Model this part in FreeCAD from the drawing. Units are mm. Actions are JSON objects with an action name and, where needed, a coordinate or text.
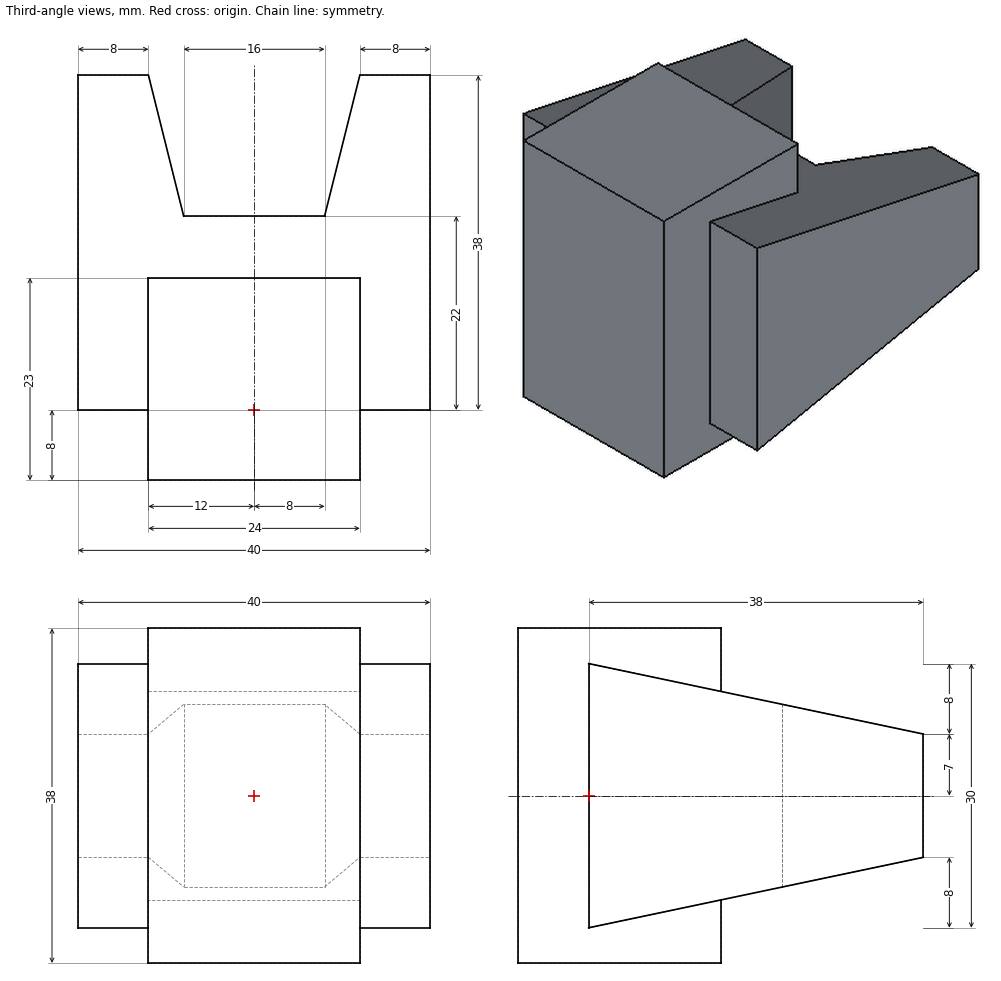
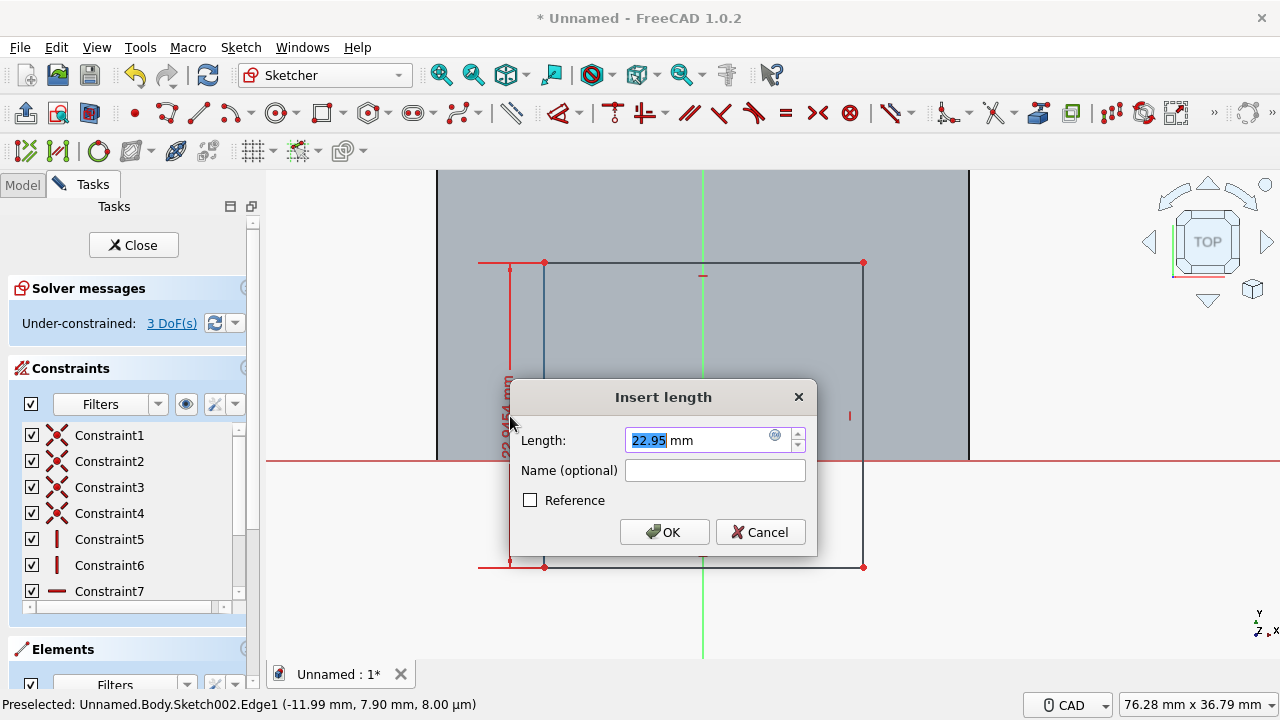
{"action": "type", "text": "23"}
{"action": "key", "text": "Return"}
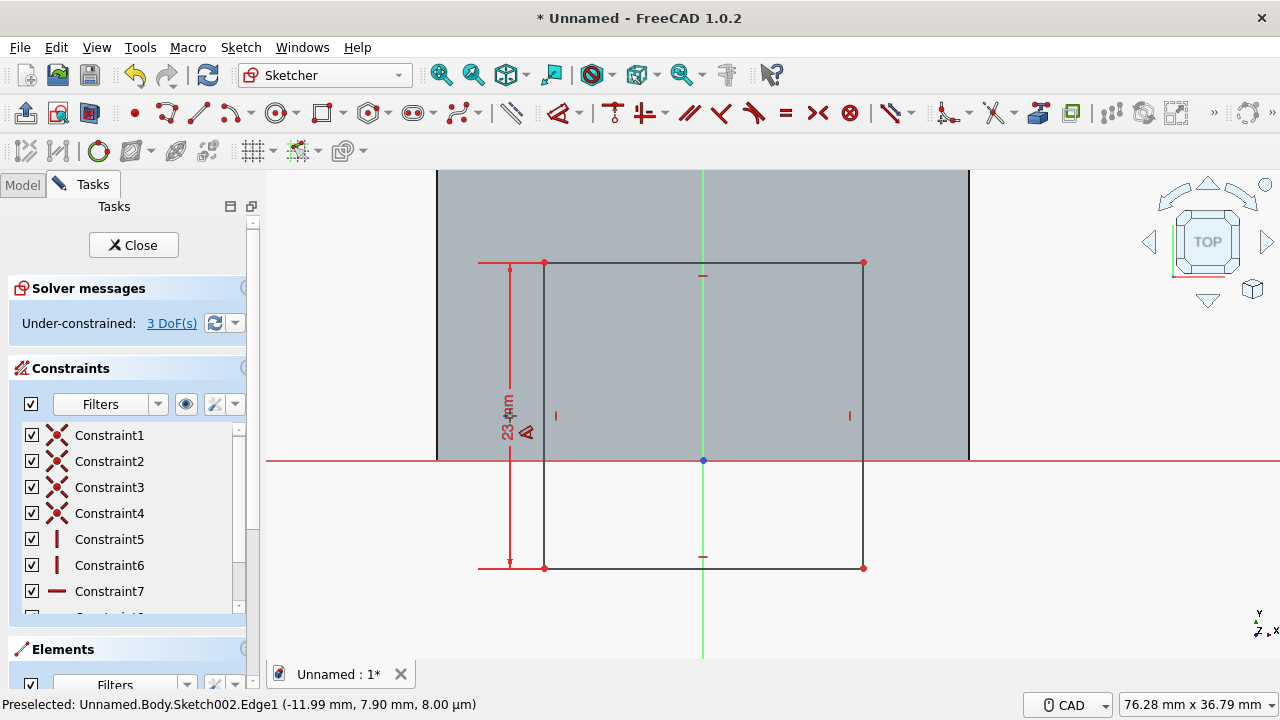
{"action": "left_click", "coordinate": [640, 569]}
{"action": "left_click", "coordinate": [630, 603]}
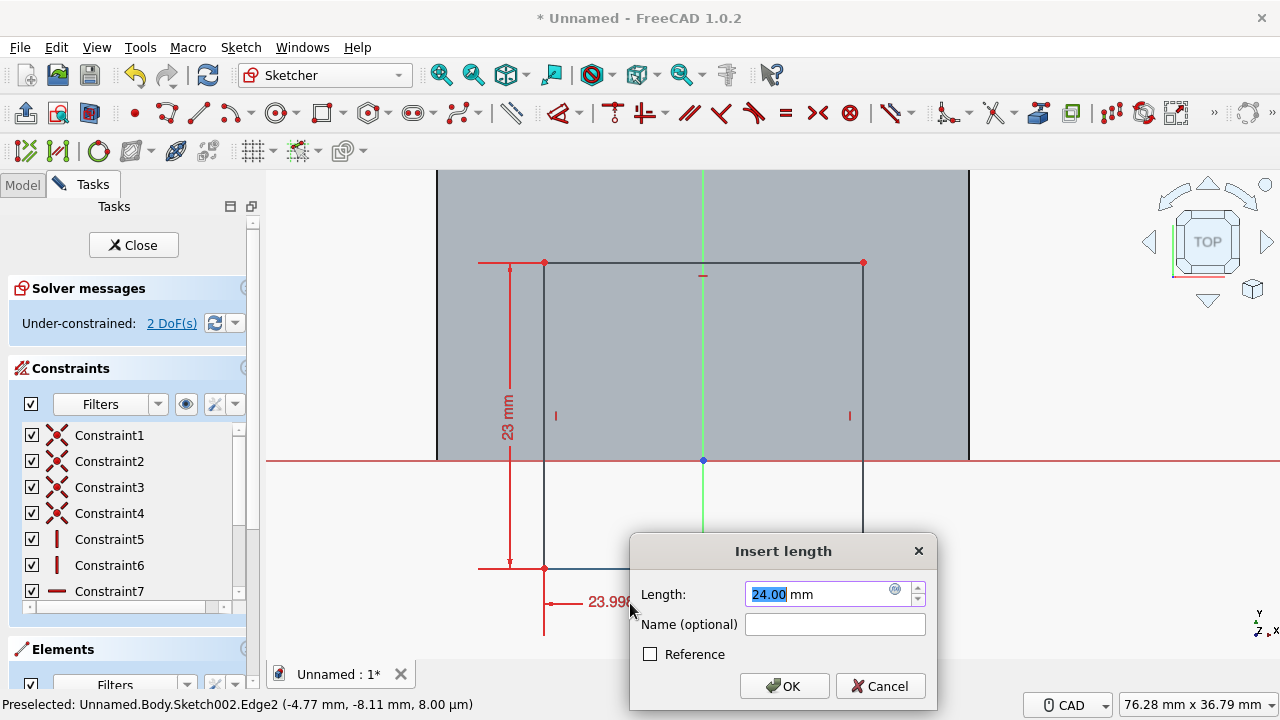
{"action": "type", "text": "24"}
{"action": "key", "text": "Return"}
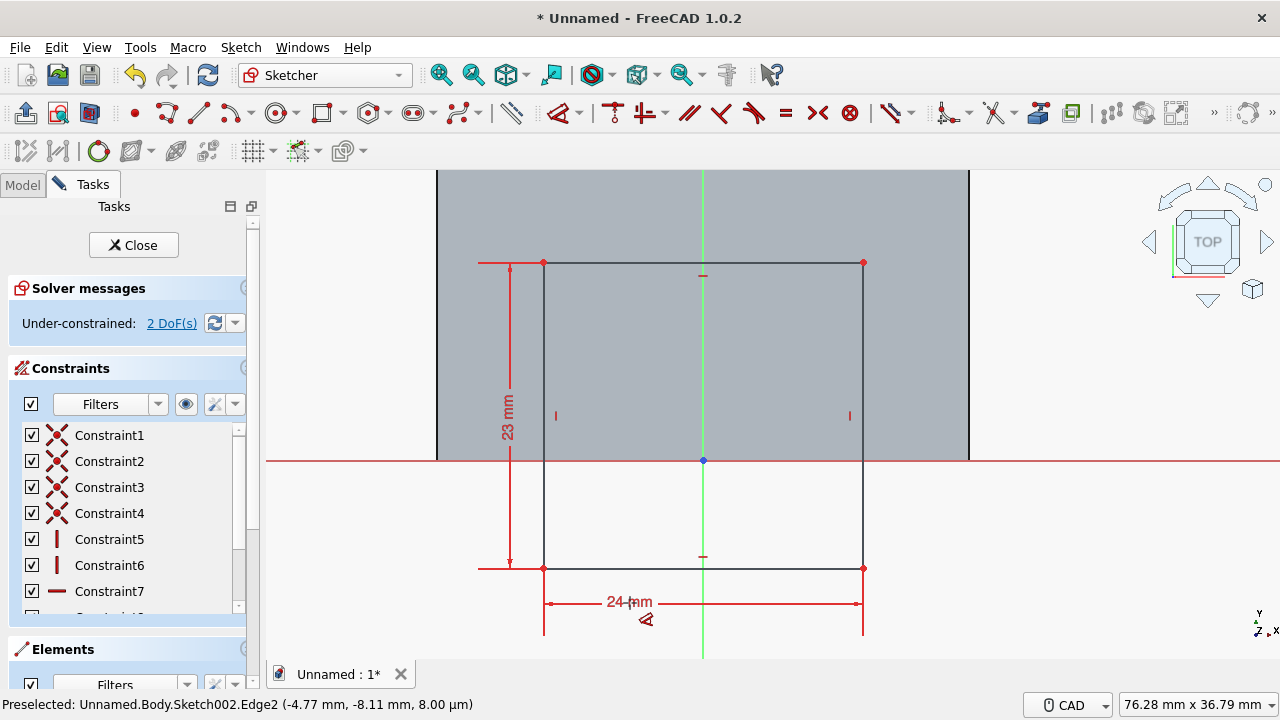
{"action": "left_click", "coordinate": [544, 569]}
{"action": "left_click", "coordinate": [510, 515]}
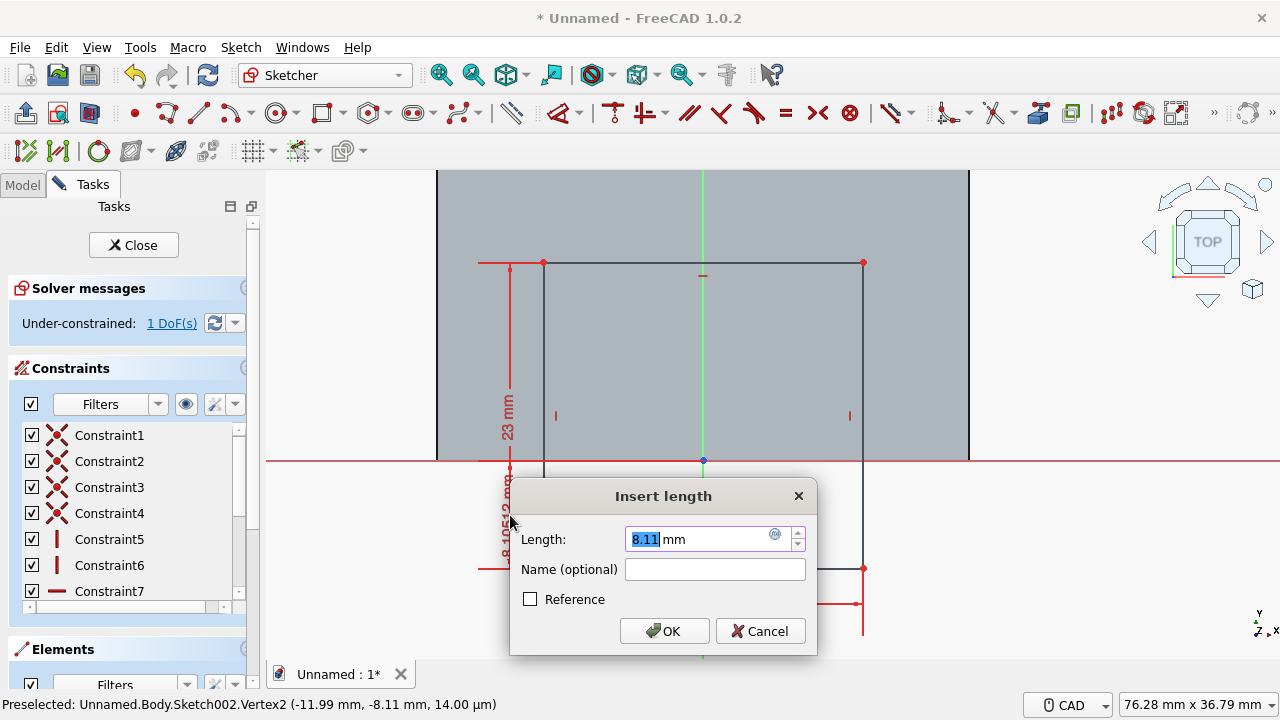
{"action": "type", "text": "8"}
{"action": "key", "text": "Return"}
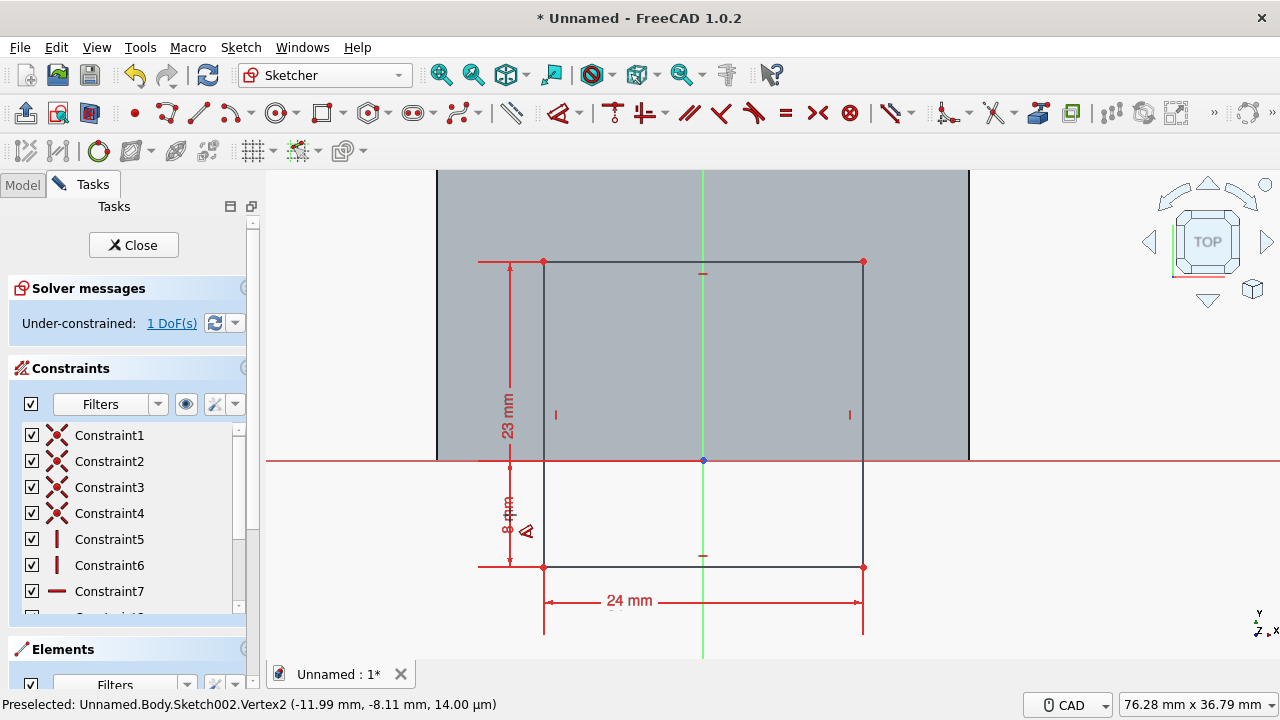
{"action": "left_click", "coordinate": [544, 262]}
{"action": "left_click", "coordinate": [624, 228]}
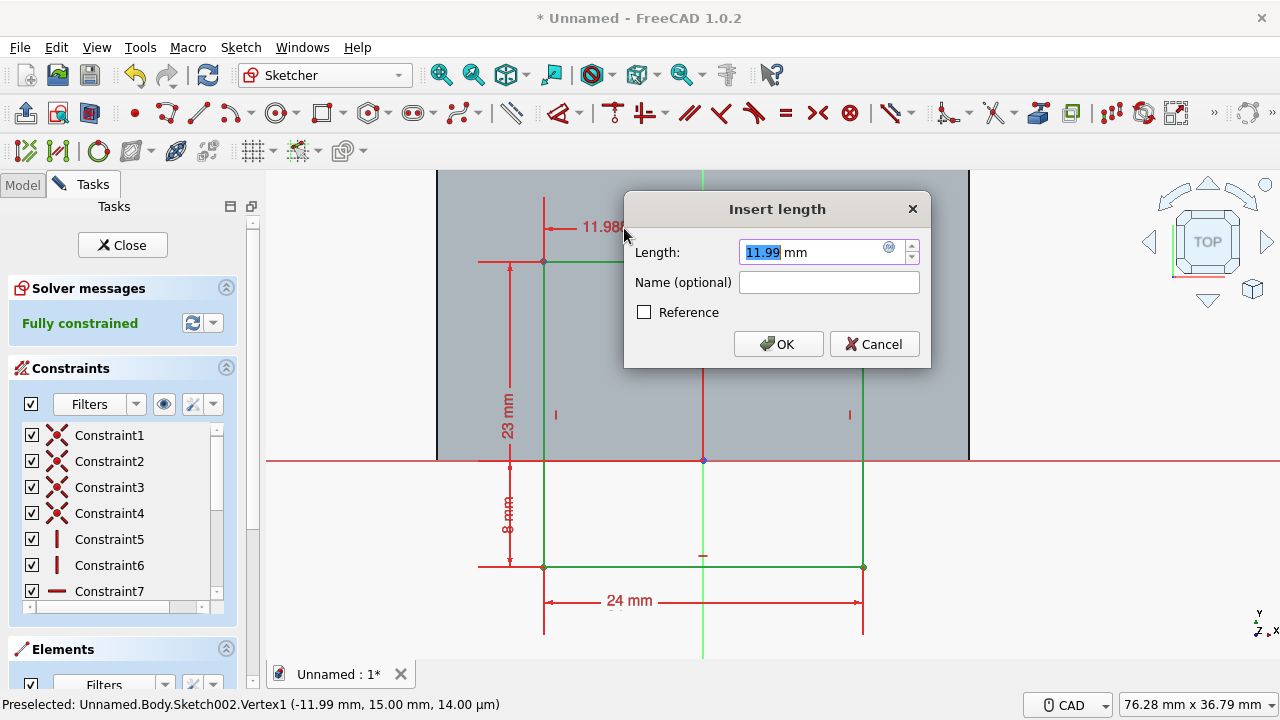
{"action": "type", "text": "12"}
{"action": "key", "text": "Return"}
{"action": "key", "text": "Escape"}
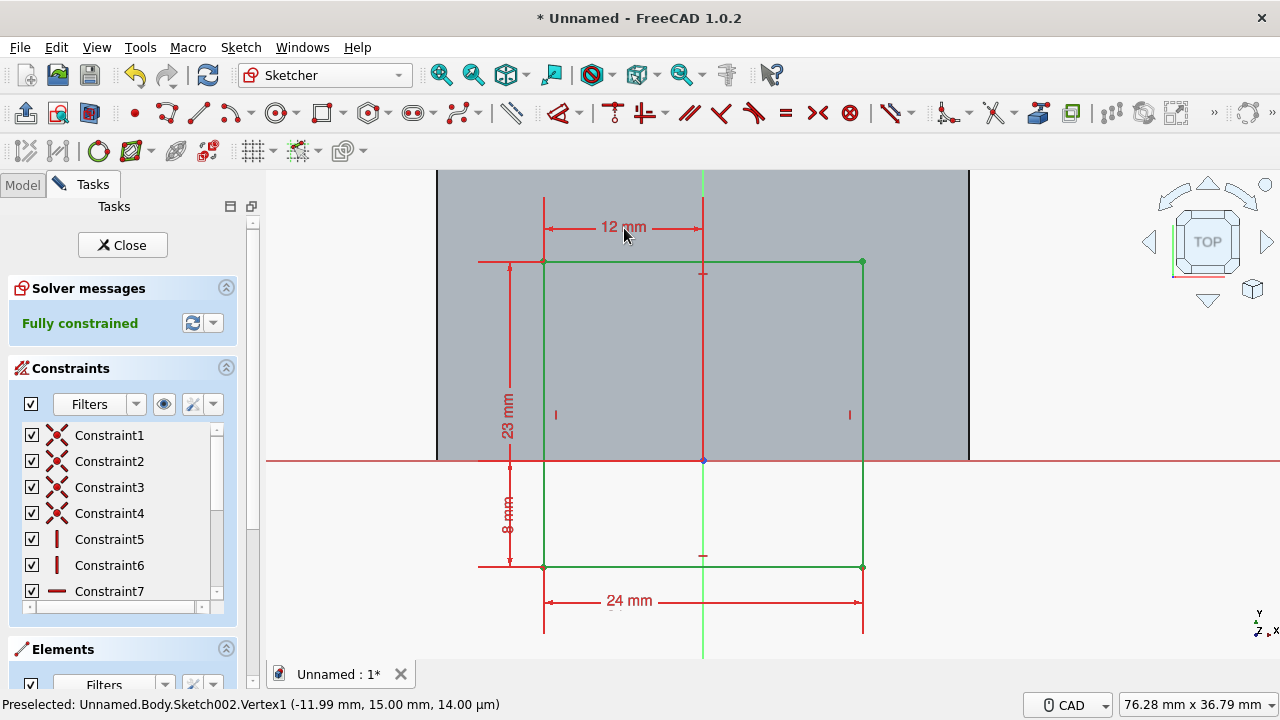
{"action": "left_click", "coordinate": [123, 245]}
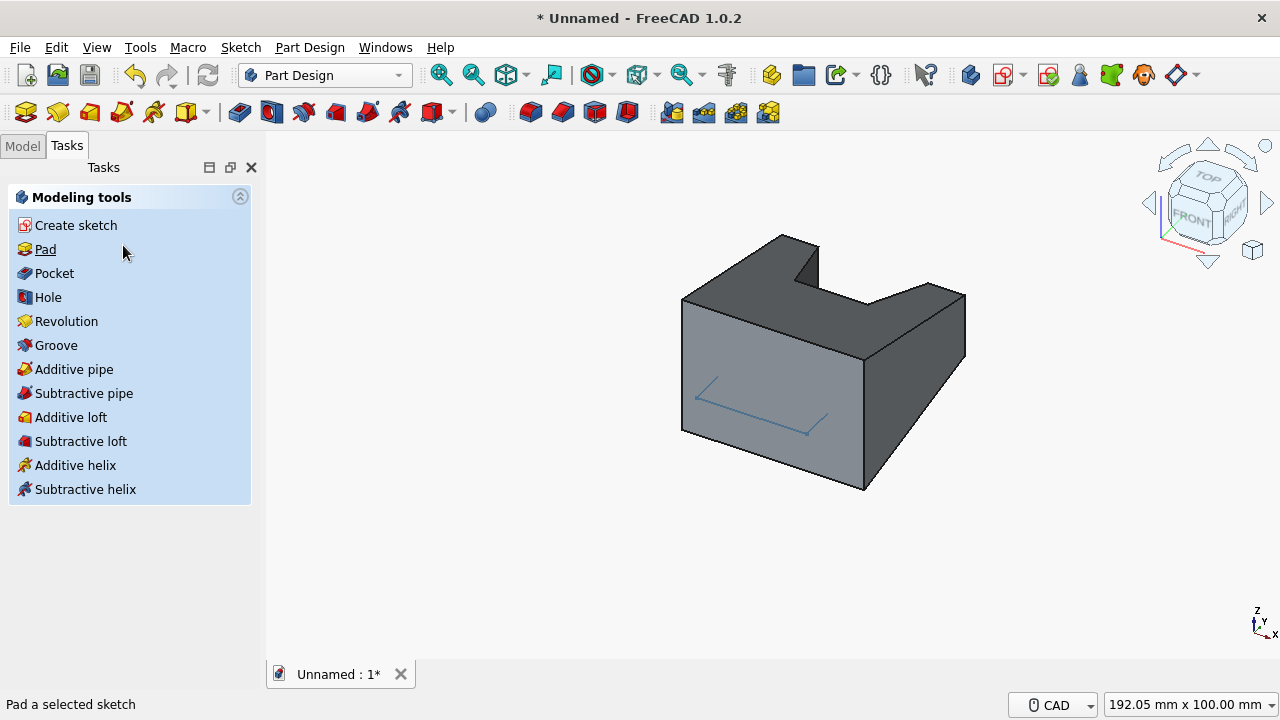
{"action": "left_click", "coordinate": [26, 112]}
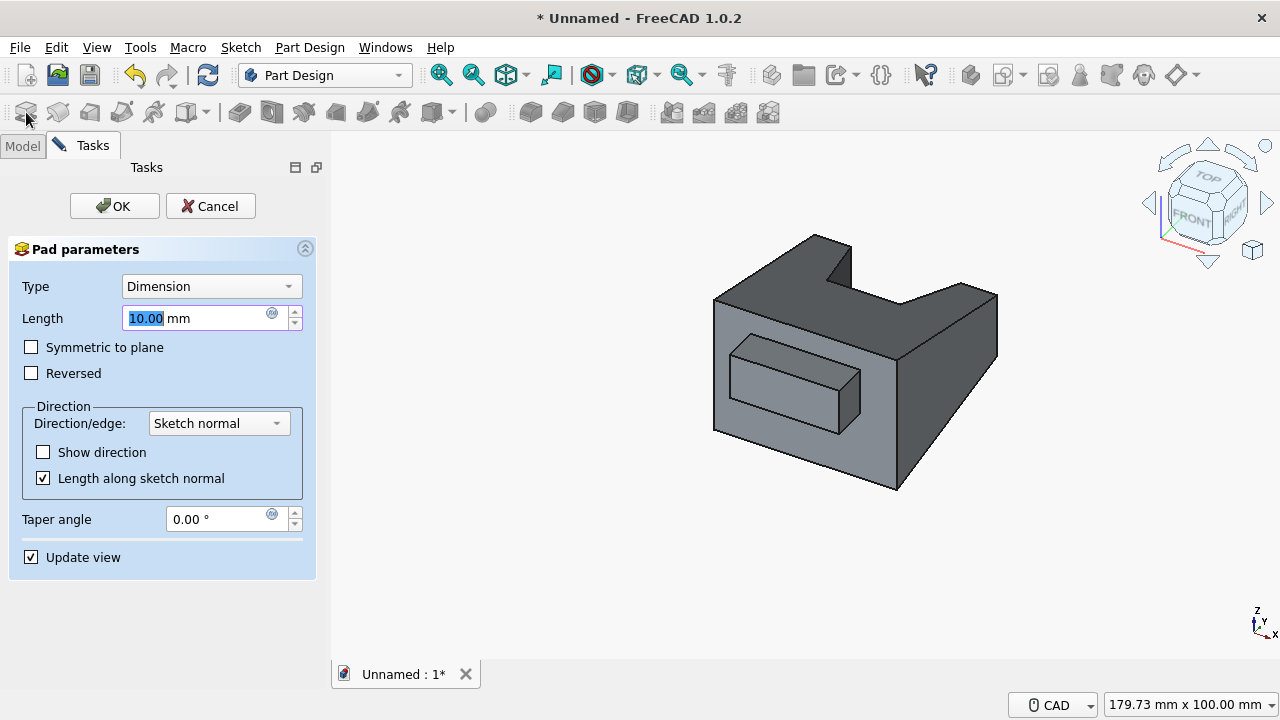
{"action": "type", "text": "38"}
{"action": "key", "text": "Tab"}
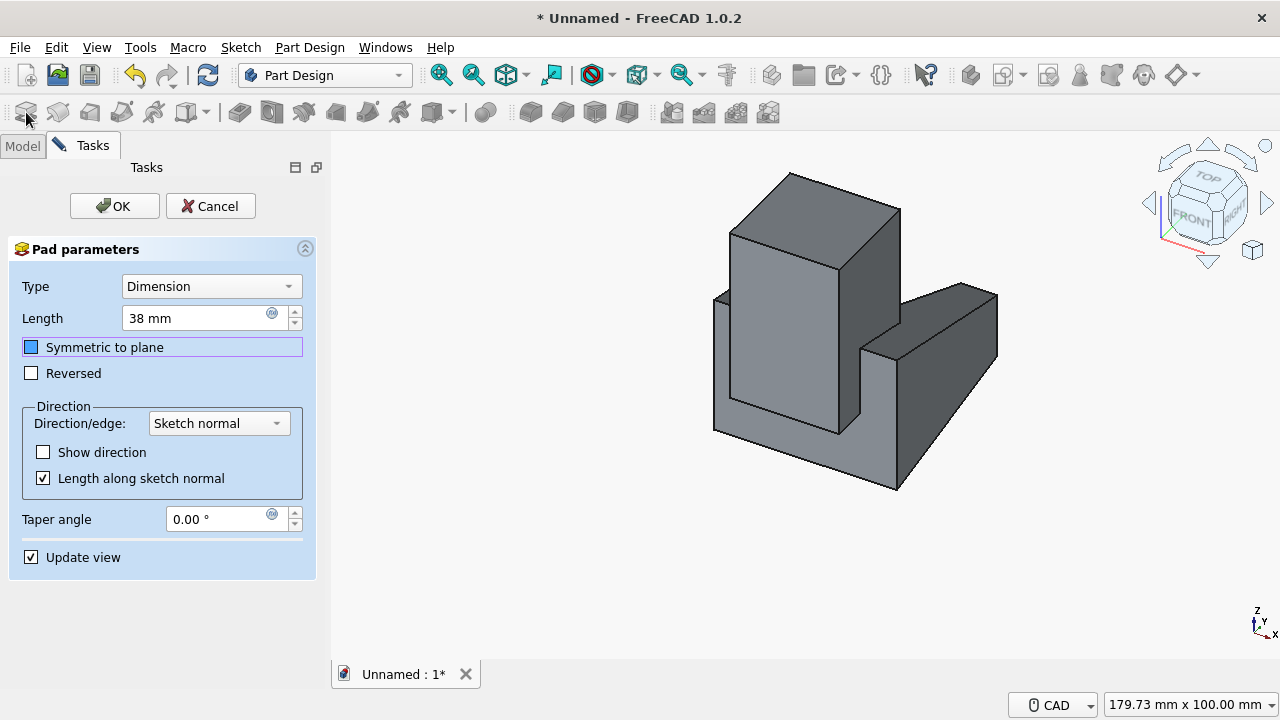
{"action": "left_click", "coordinate": [30, 347]}